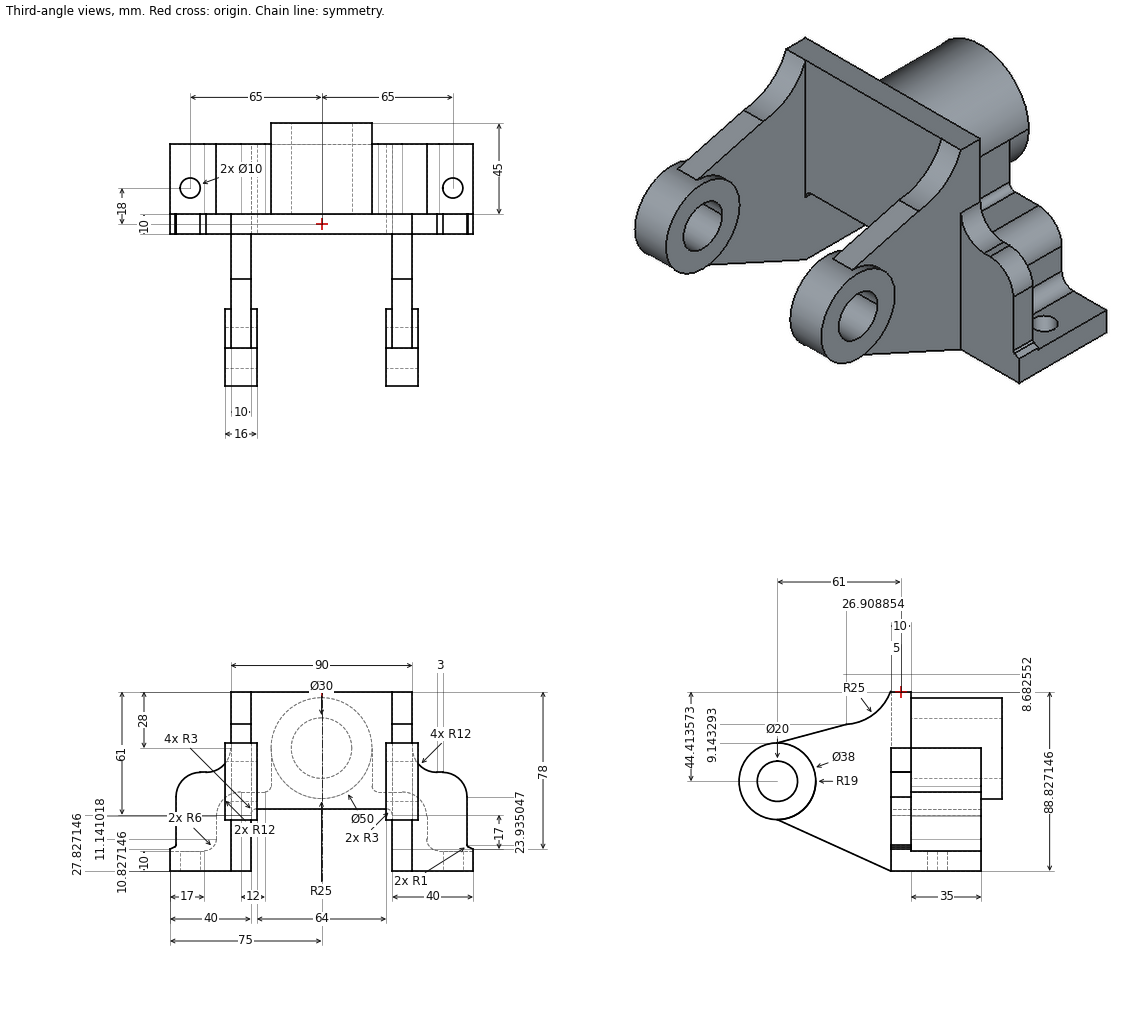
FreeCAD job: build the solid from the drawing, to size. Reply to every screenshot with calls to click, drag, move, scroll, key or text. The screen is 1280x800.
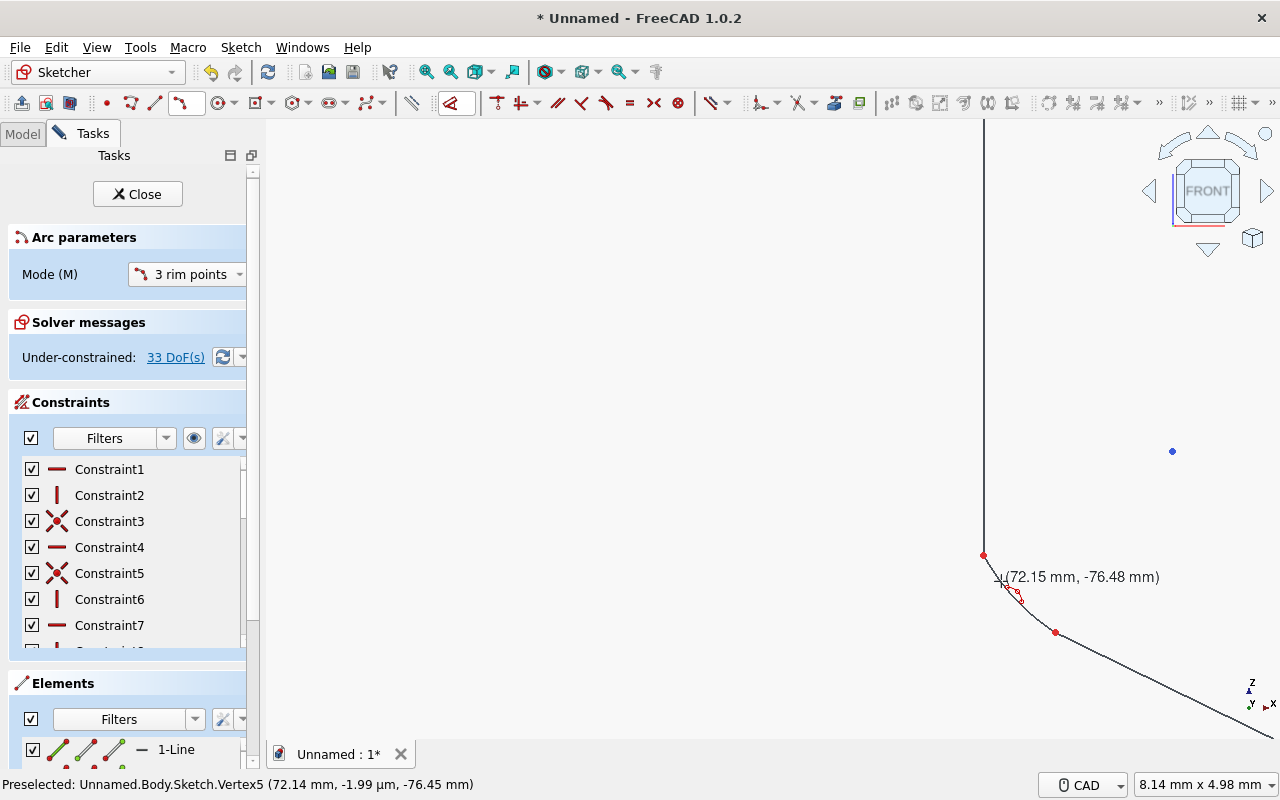
scroll(1074, 621, down, 16)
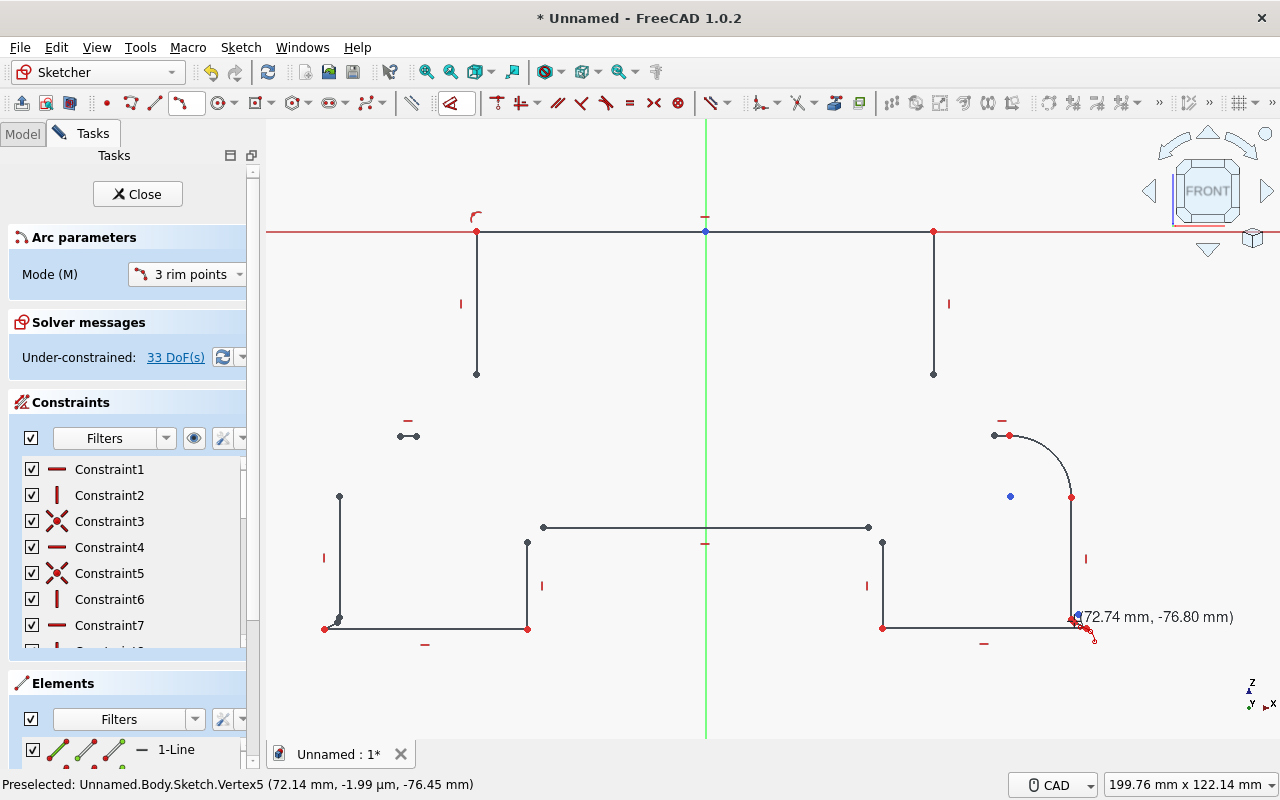
click(883, 542)
click(868, 528)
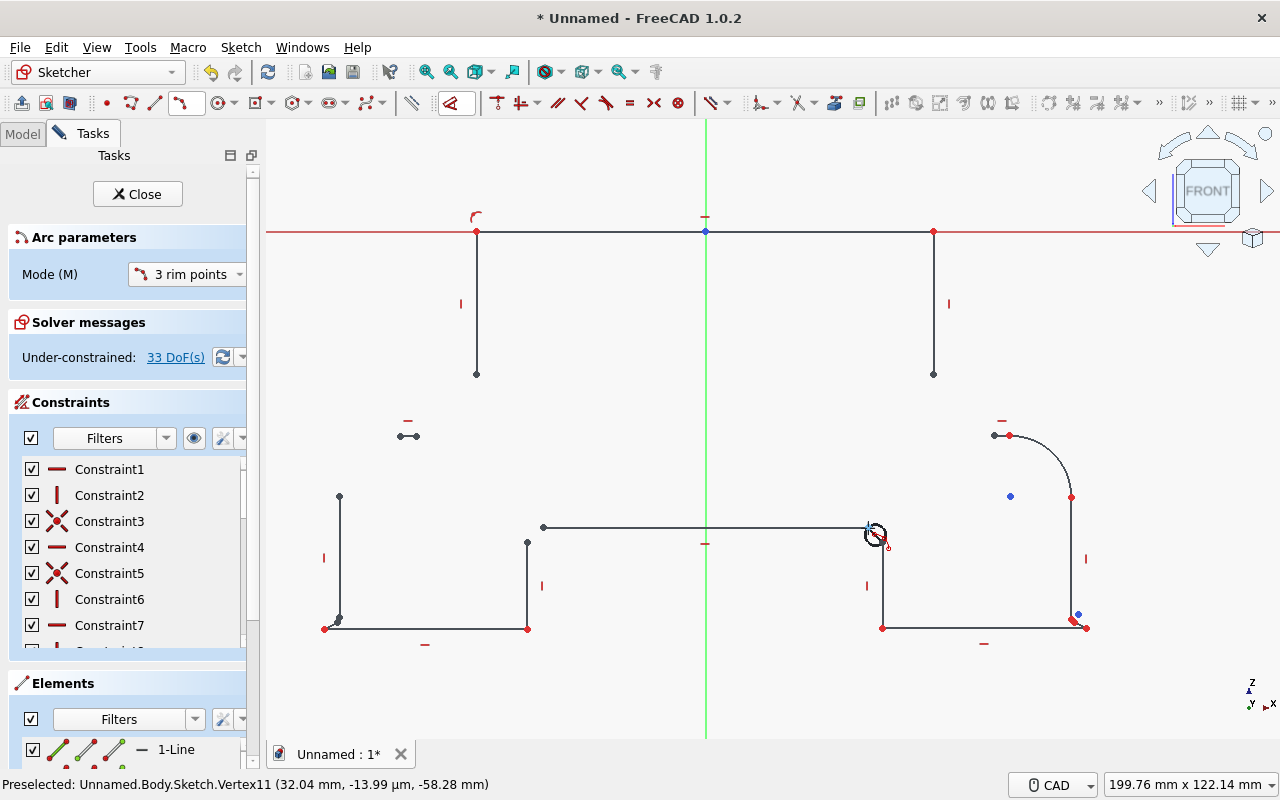
scroll(879, 531, up, 7)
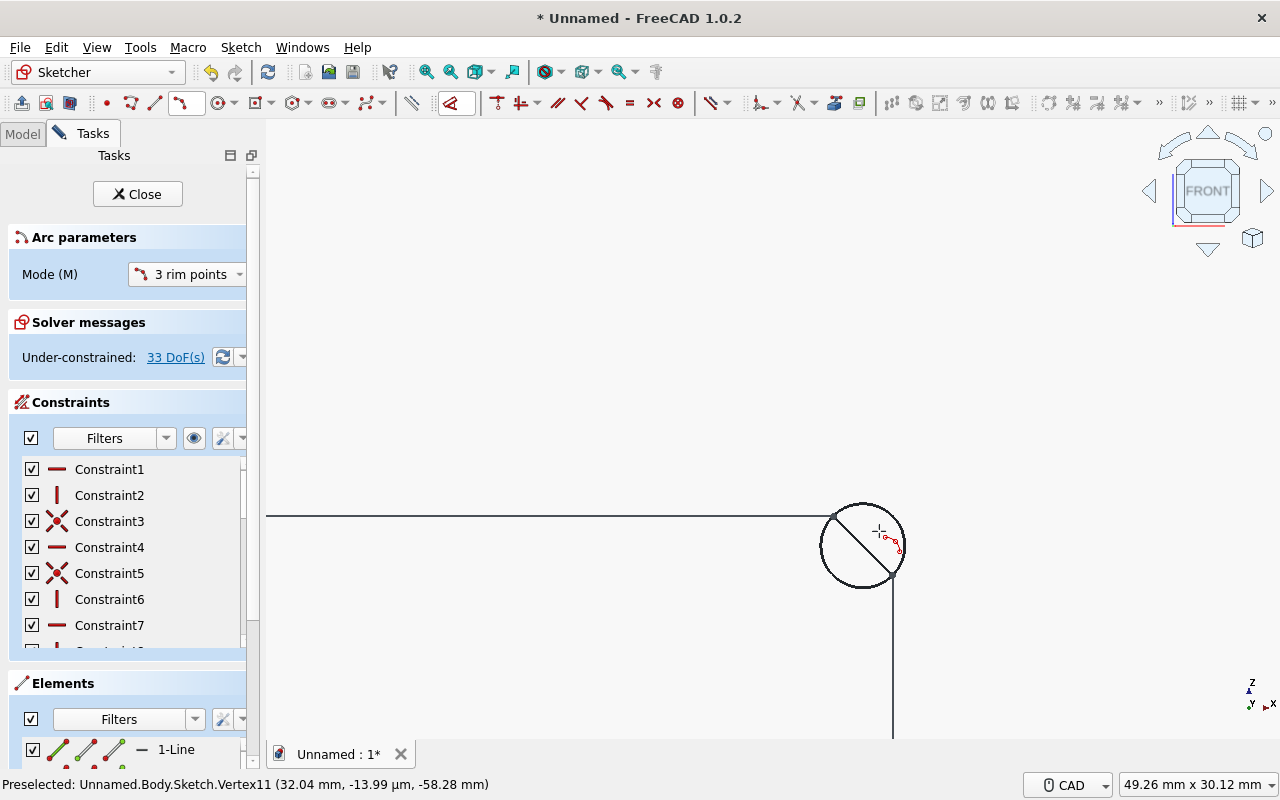
click(876, 528)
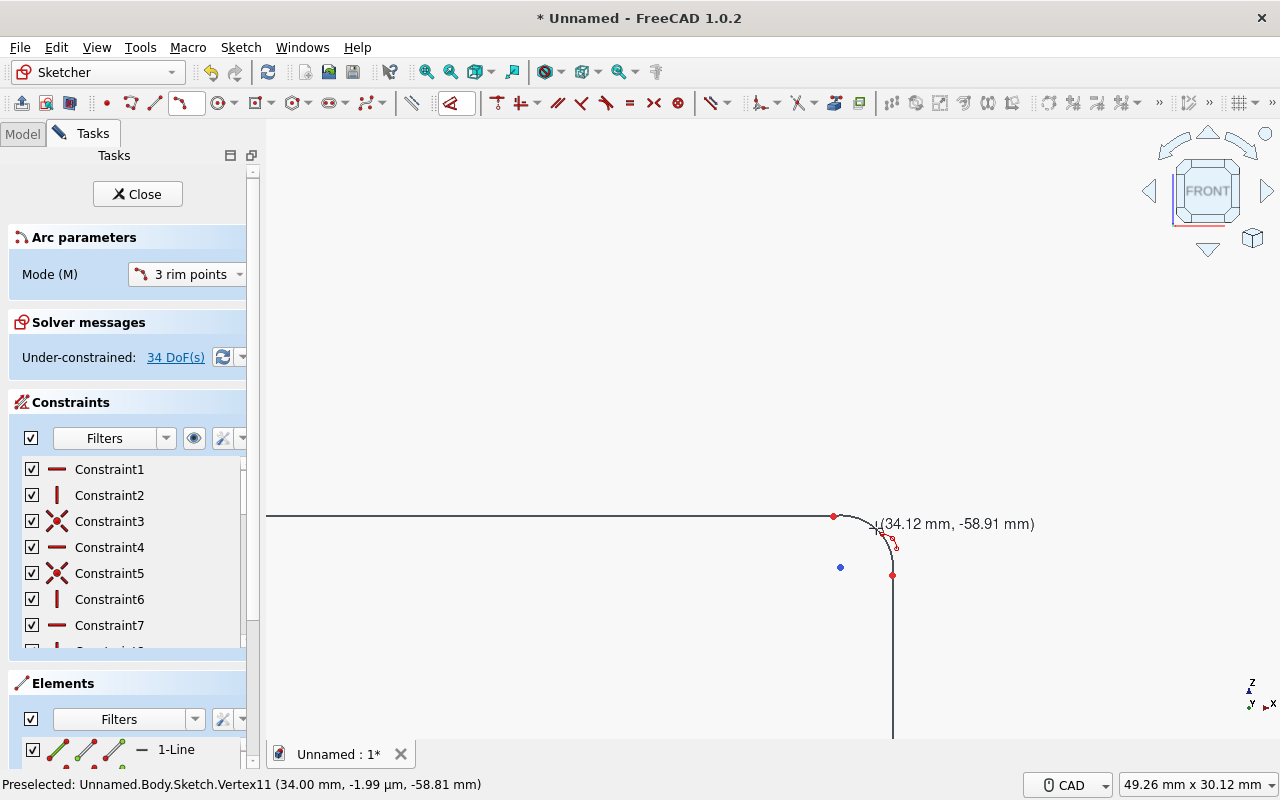
scroll(839, 507, down, 8)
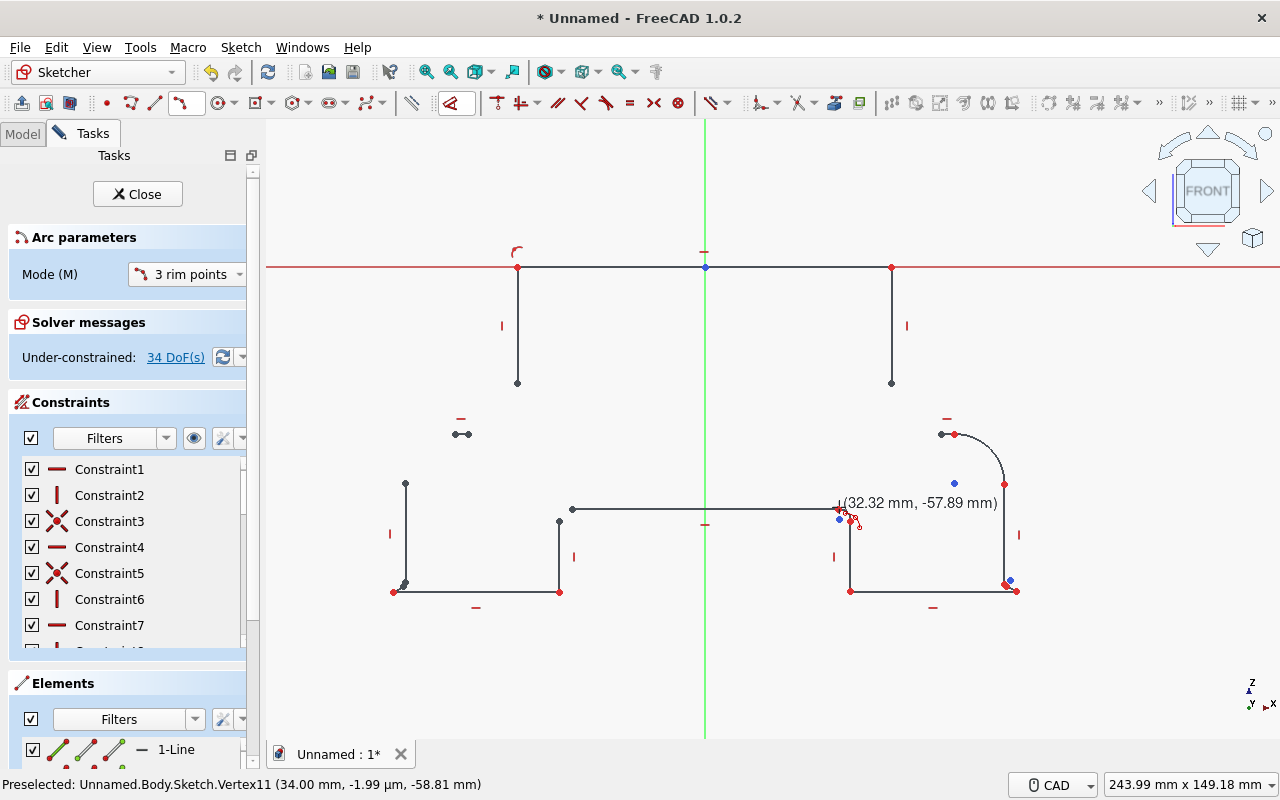
click(572, 509)
click(559, 521)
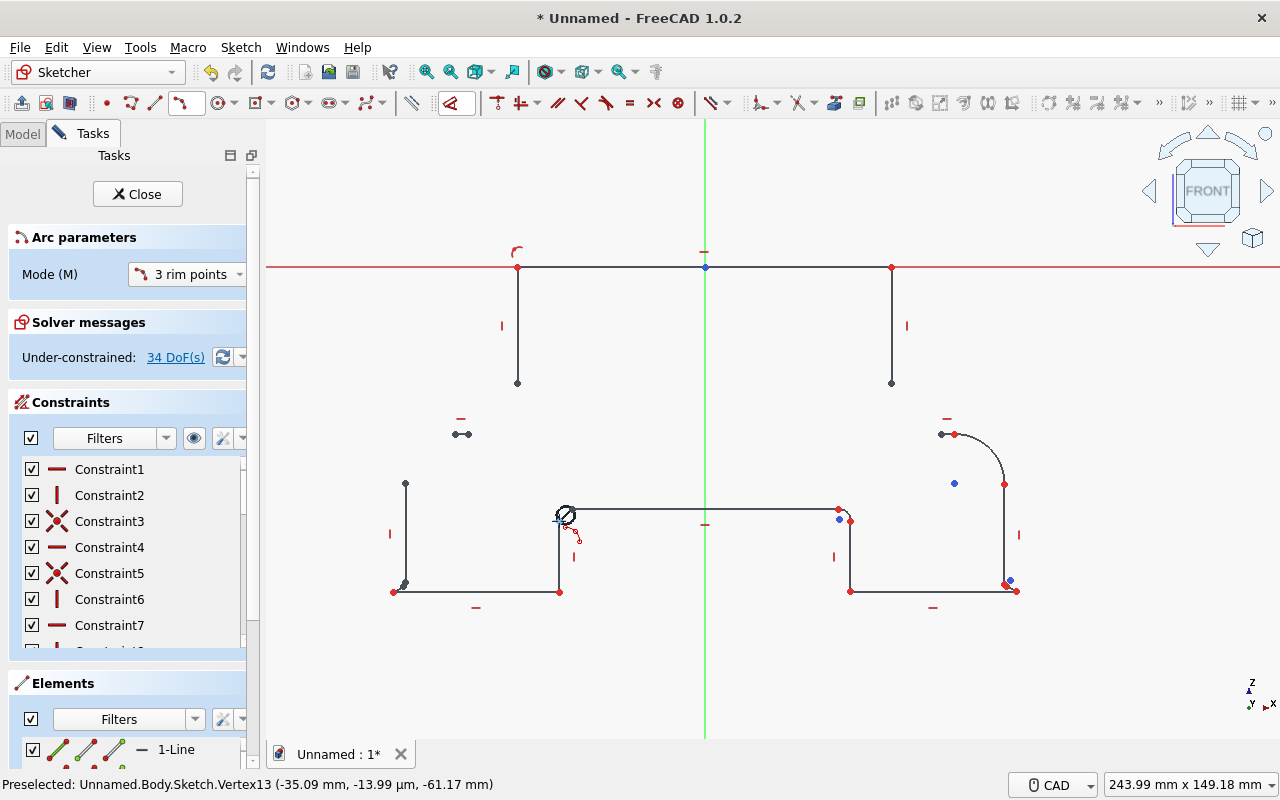
scroll(563, 512, up, 8)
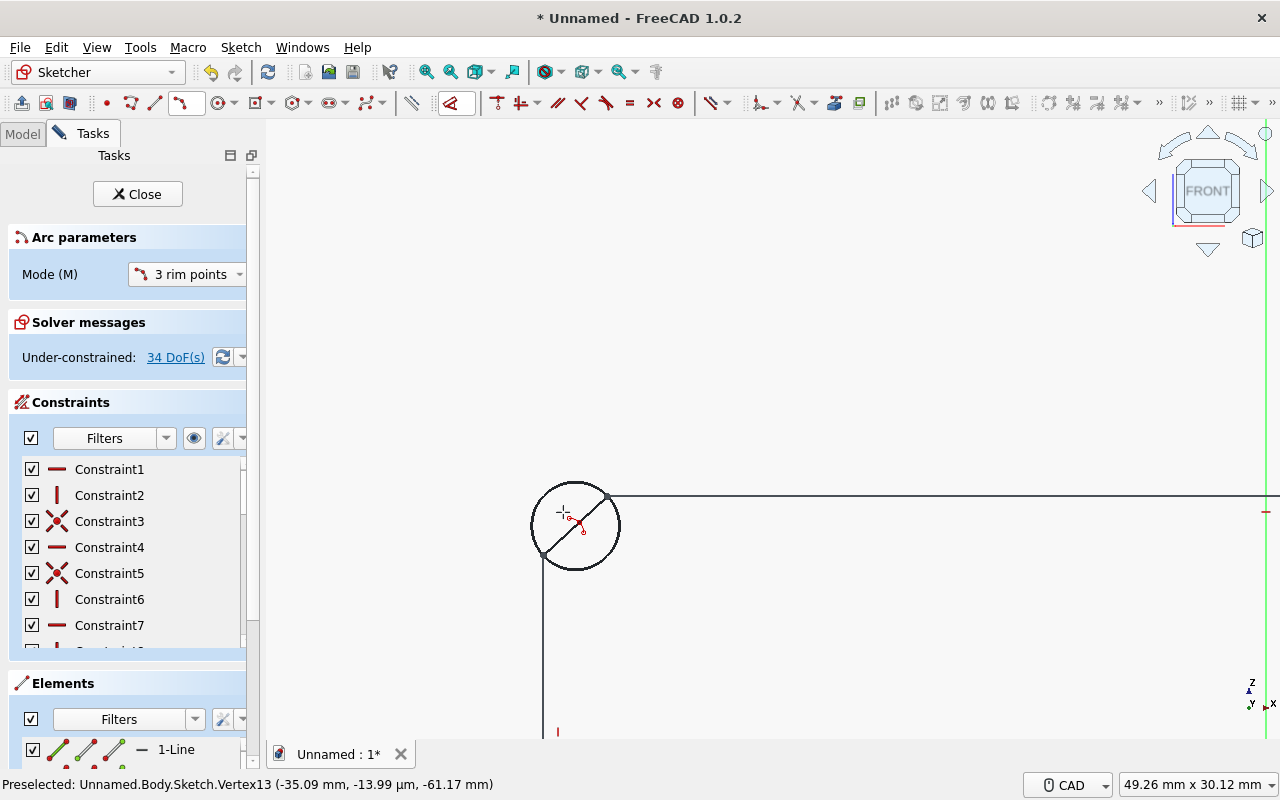
click(563, 509)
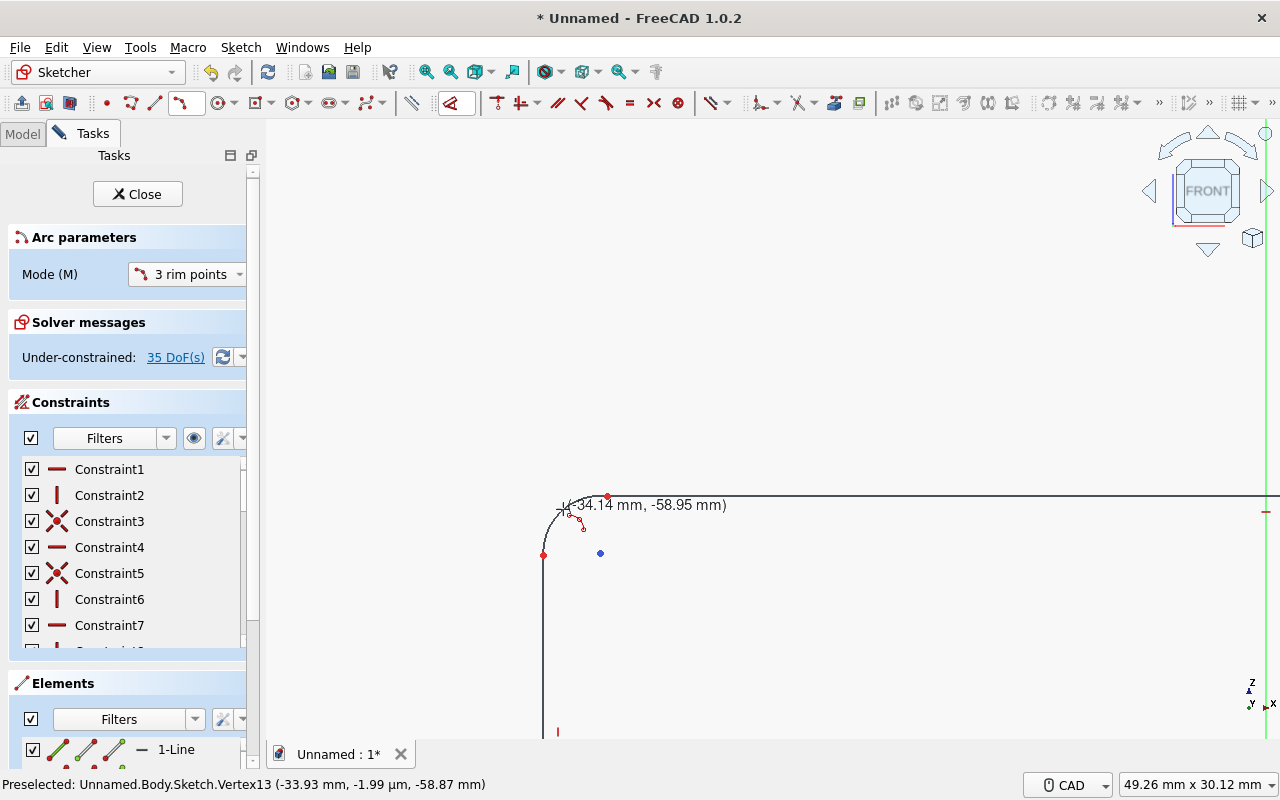
scroll(563, 512, down, 8)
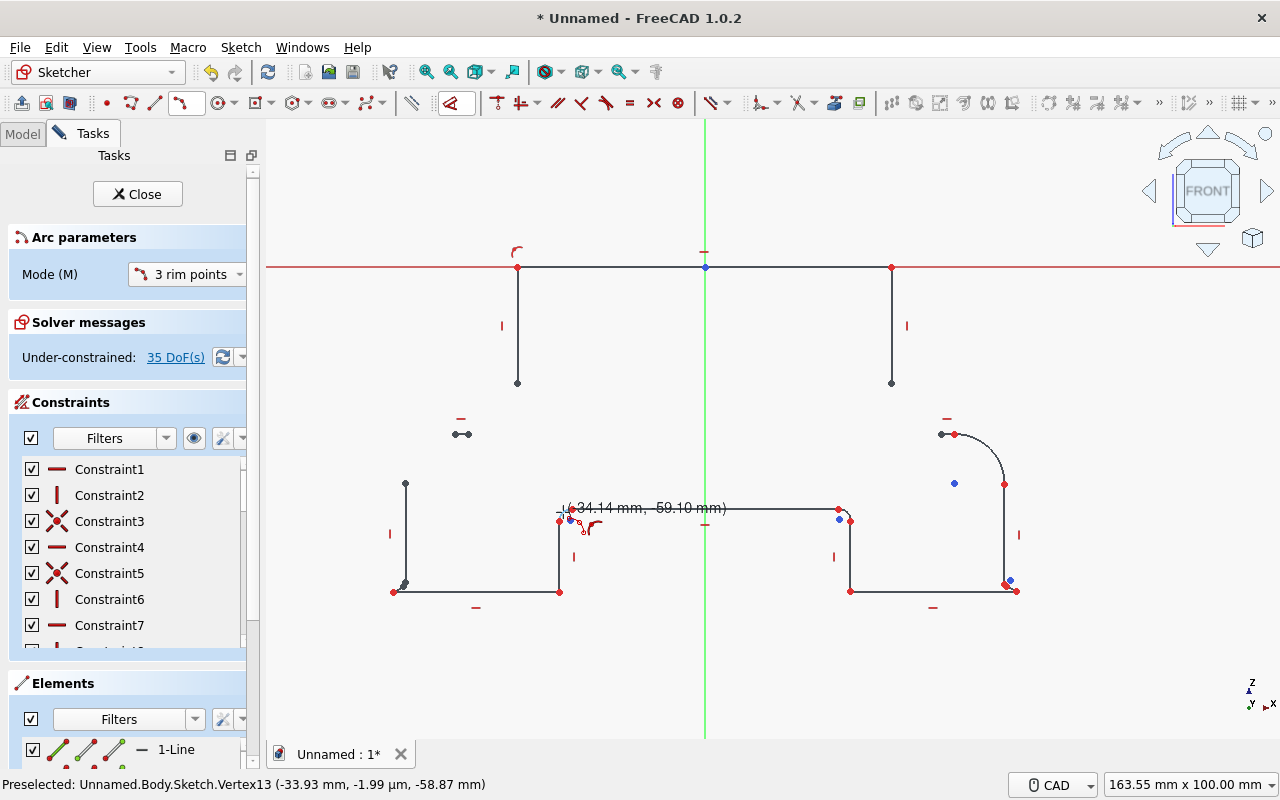
scroll(404, 586, up, 7)